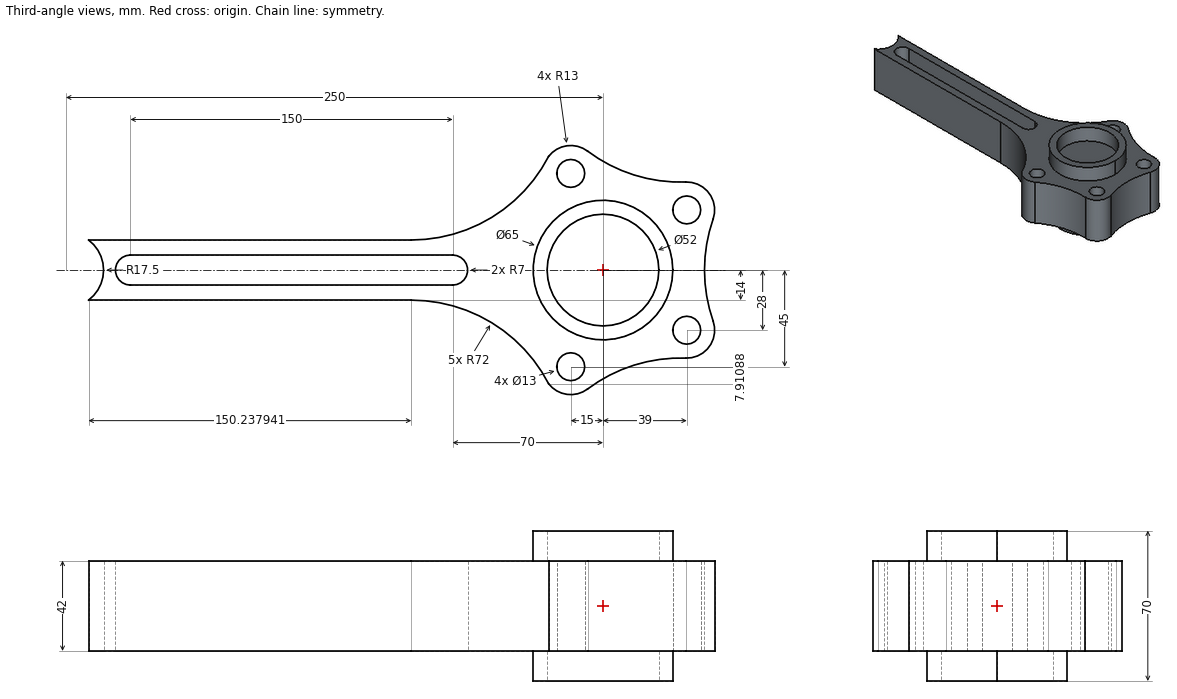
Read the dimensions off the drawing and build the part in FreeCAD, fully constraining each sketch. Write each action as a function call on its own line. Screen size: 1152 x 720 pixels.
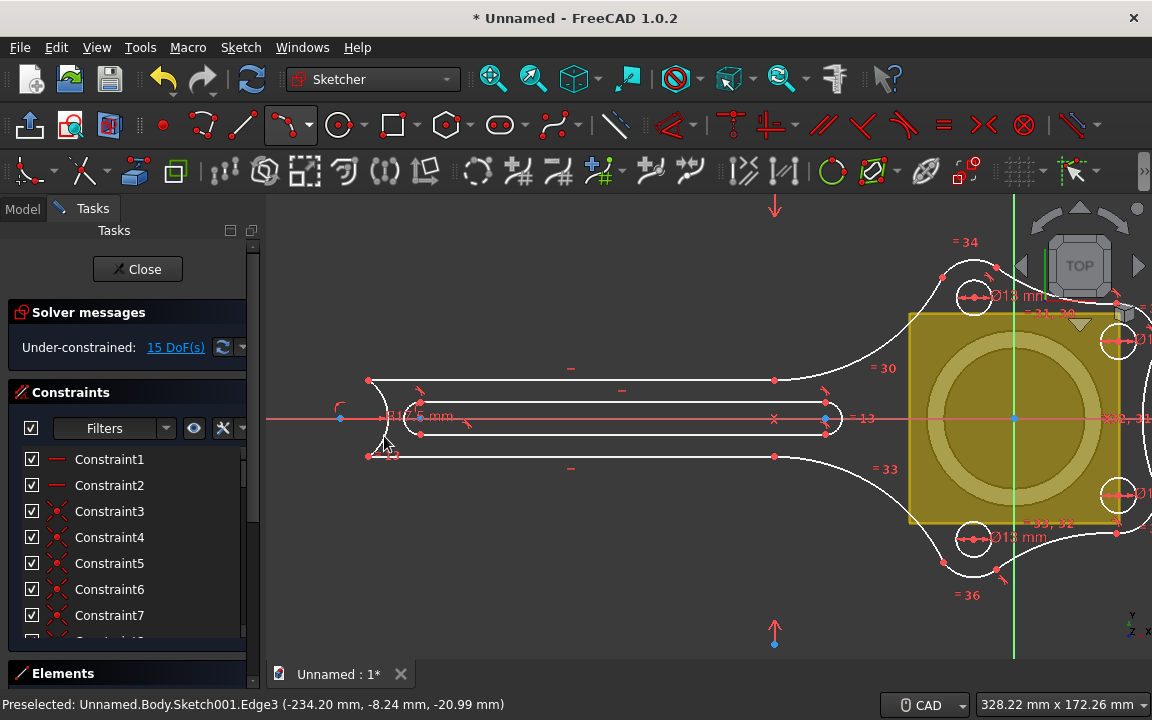
click(835, 370)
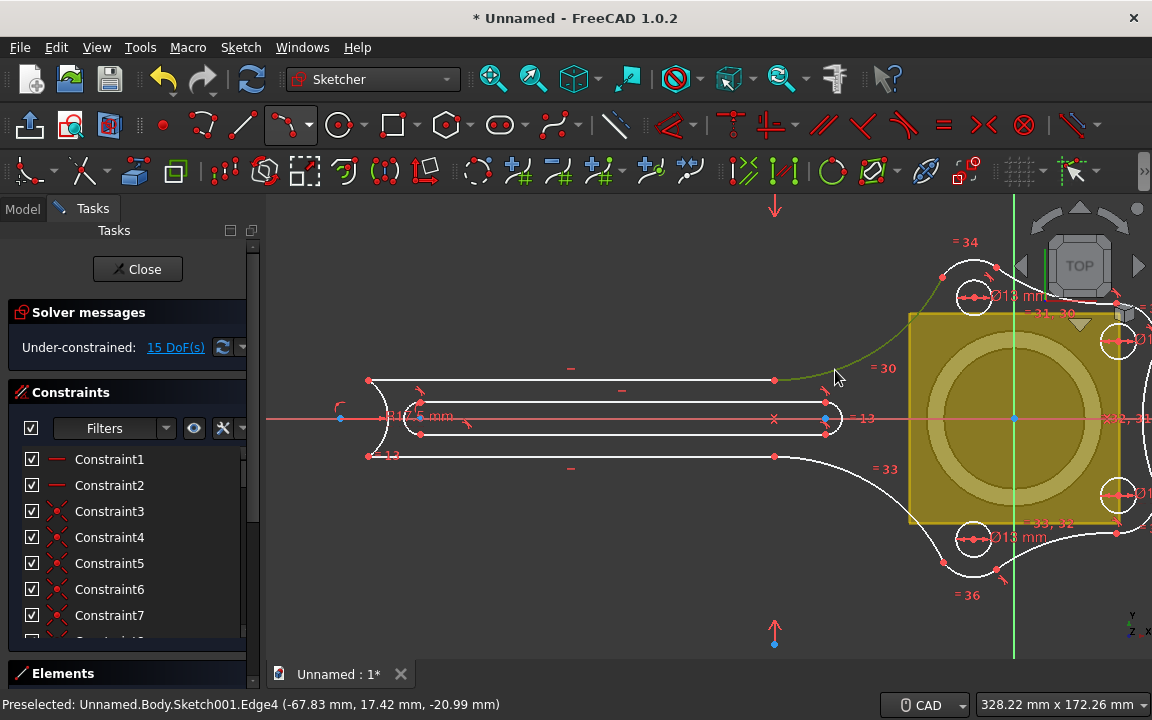
click(696, 126)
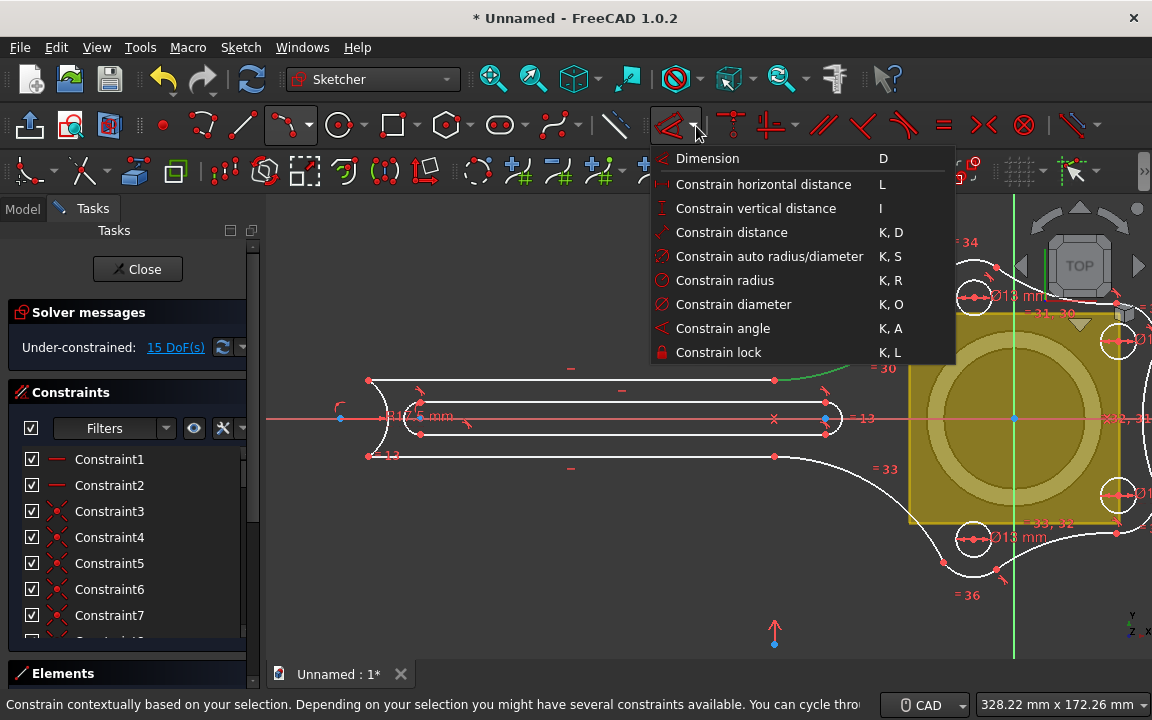
click(803, 280)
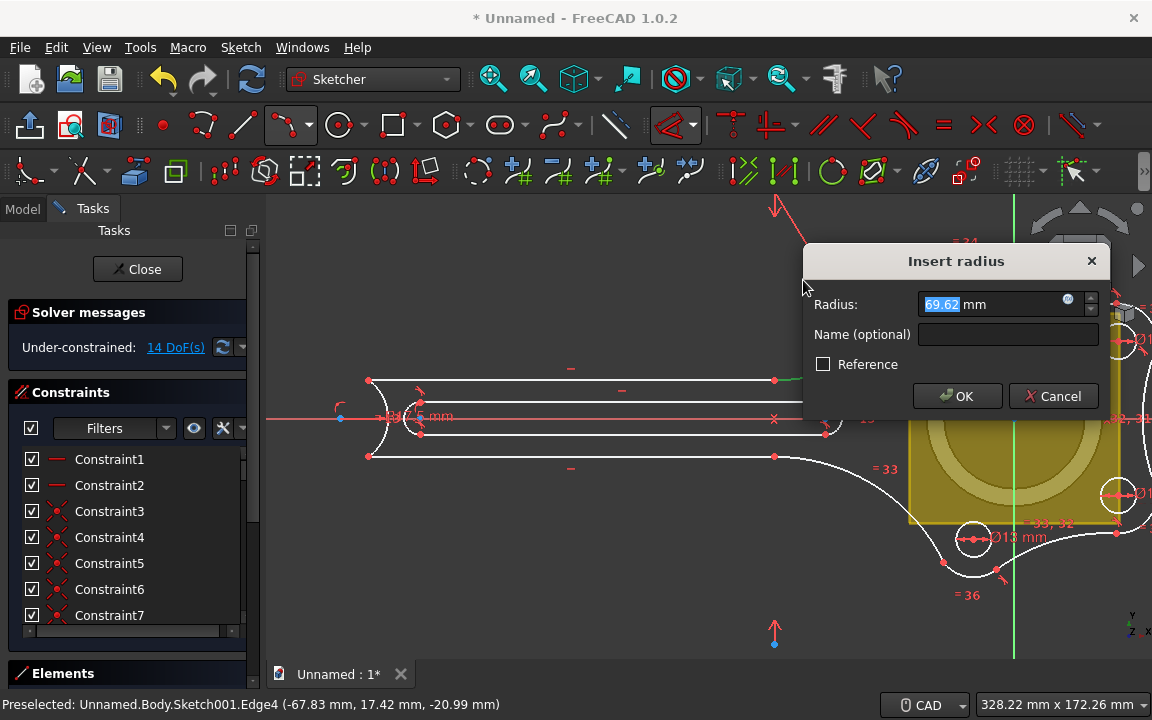
text(72)
key(Return)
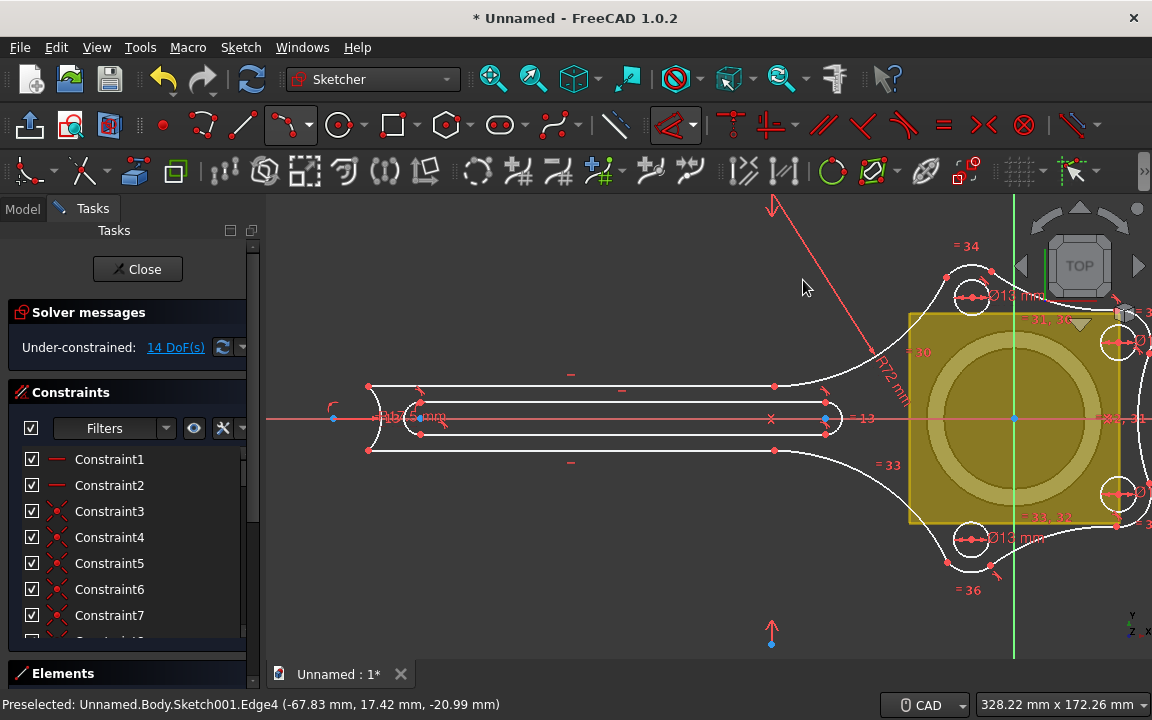
click(978, 266)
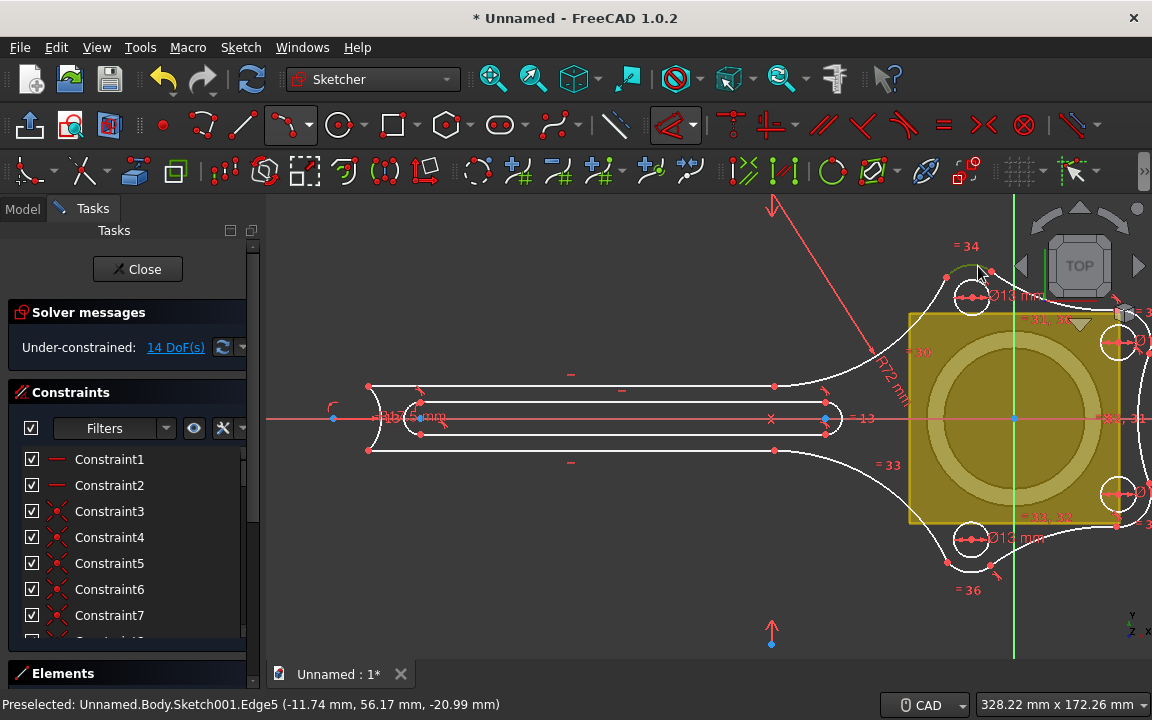
key(k)
key(r)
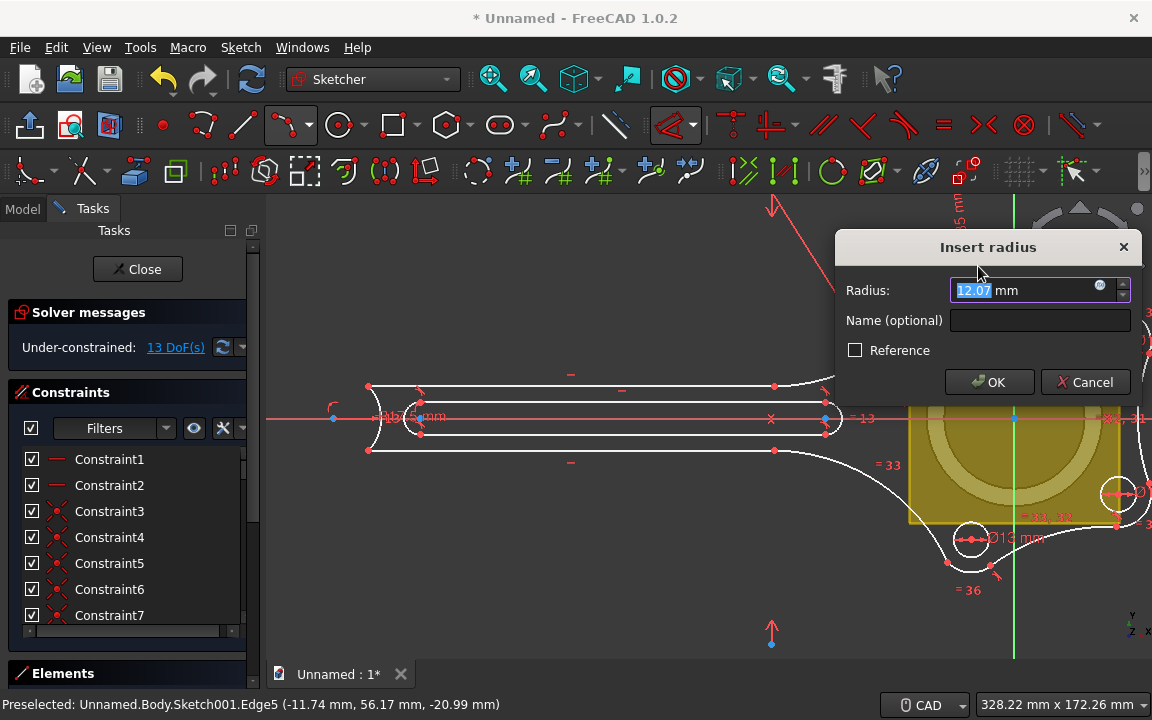
text(13)
key(Return)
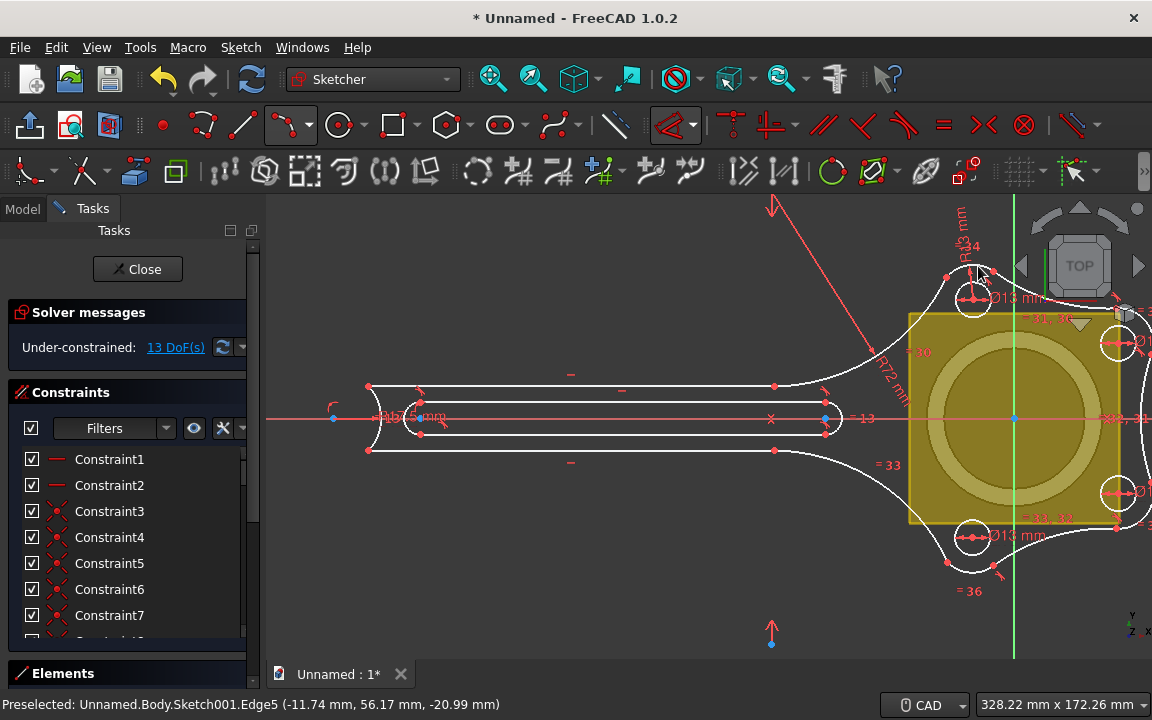
scroll(407, 409, up, 4)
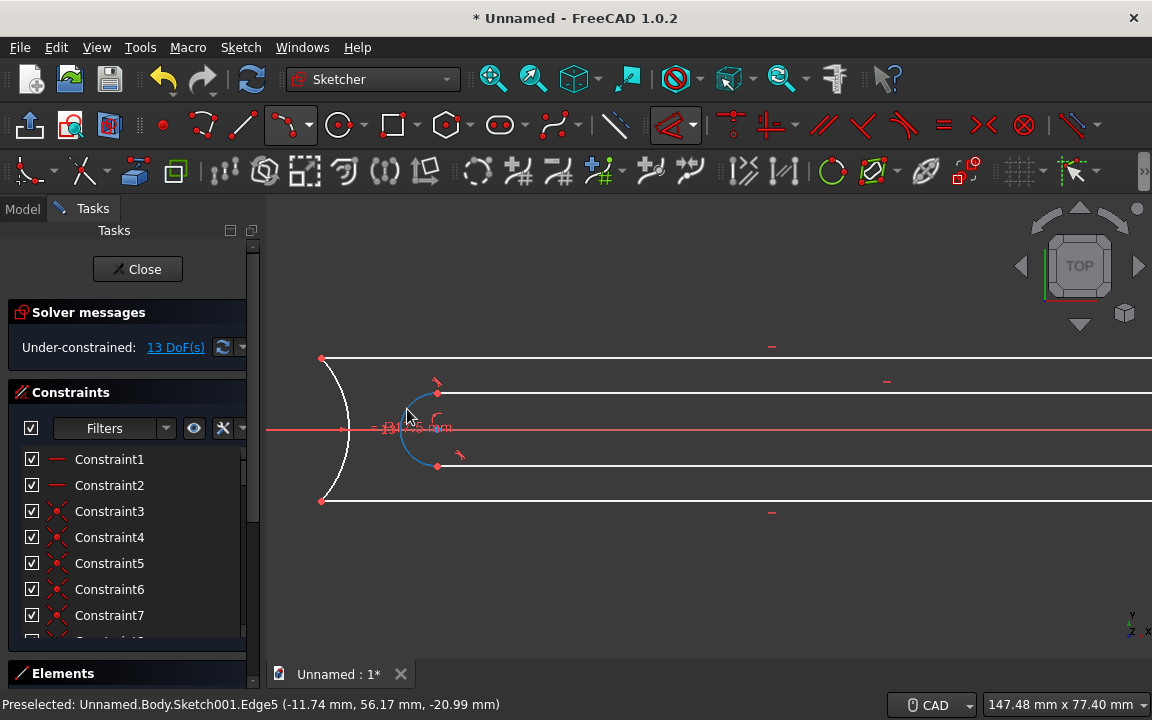
click(407, 408)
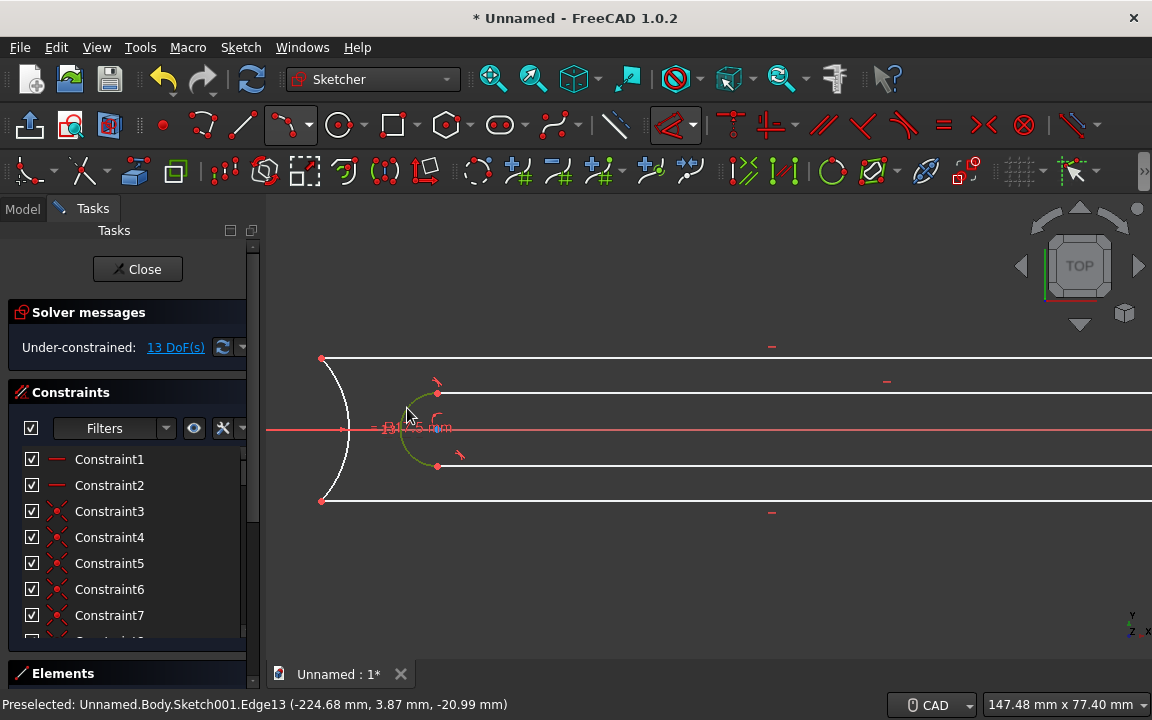
key(k)
key(r)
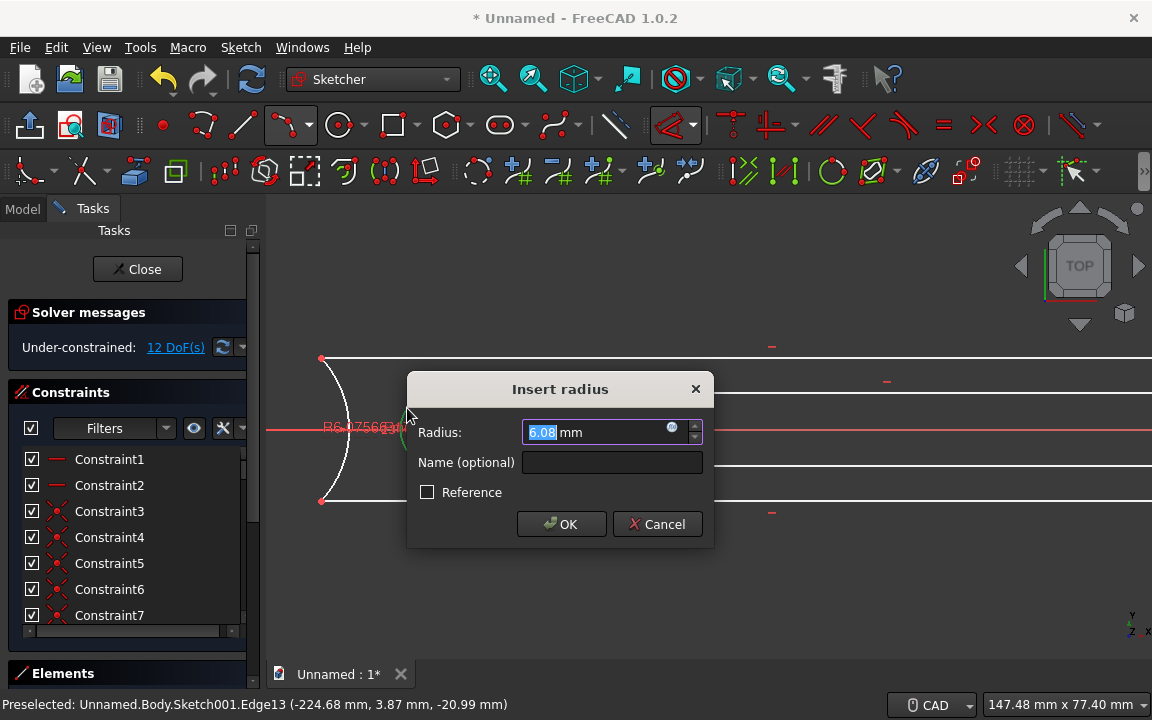
text(7)
key(Return)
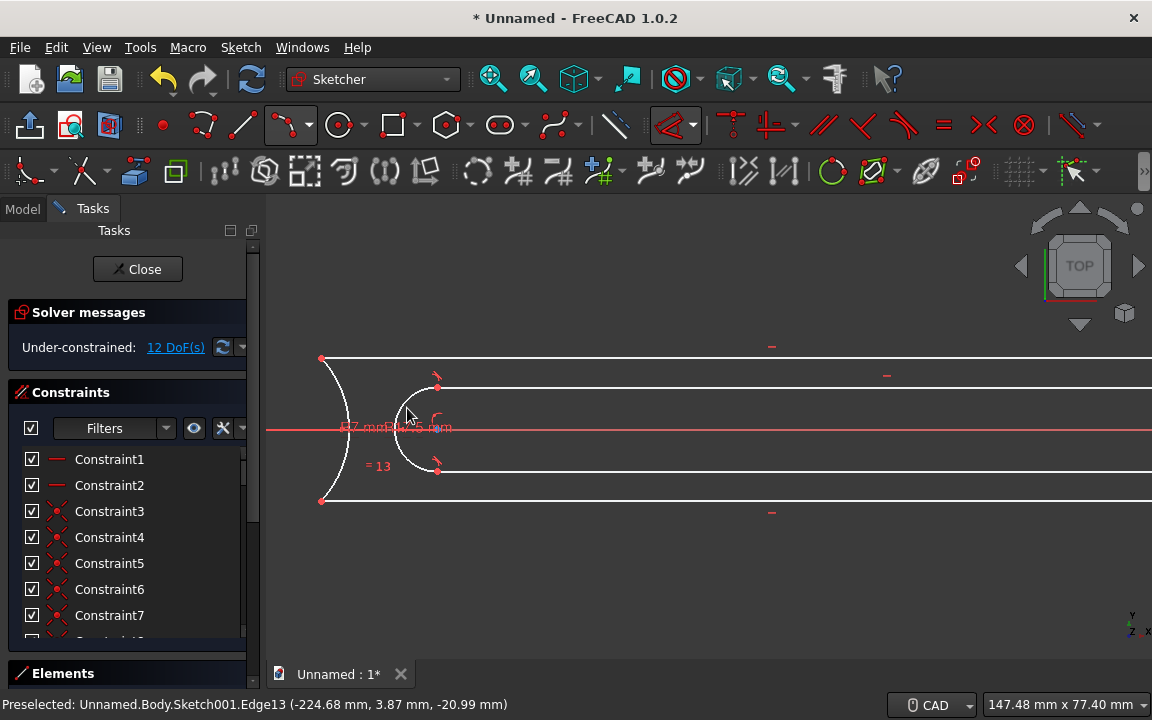
scroll(402, 425, down, 6)